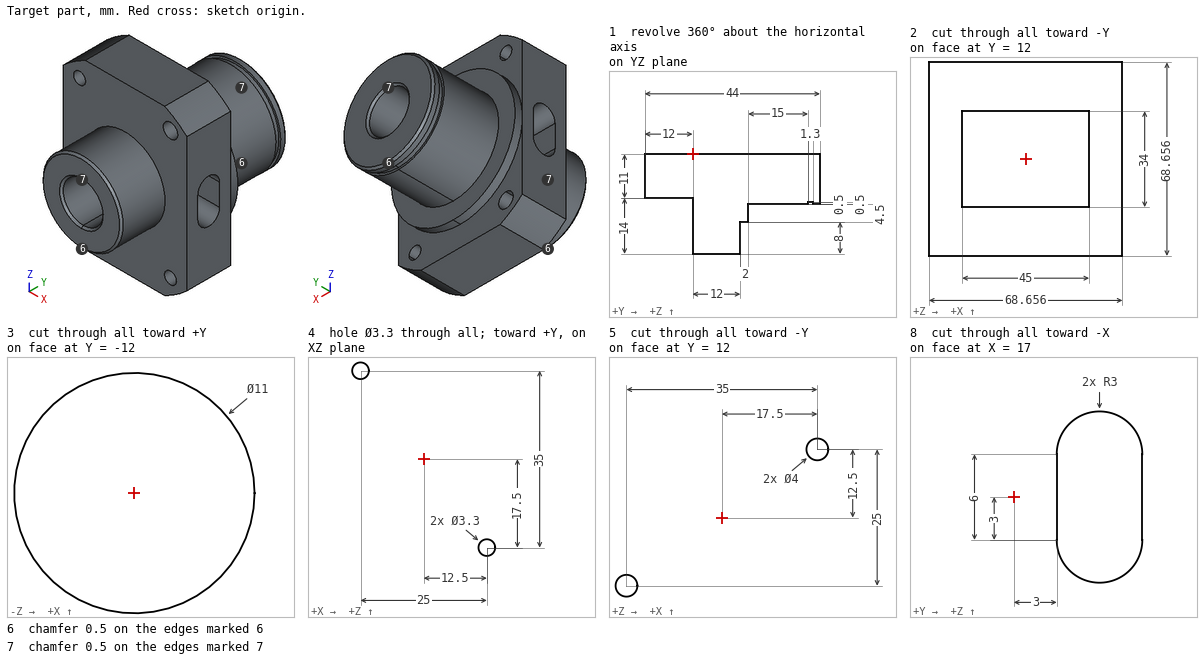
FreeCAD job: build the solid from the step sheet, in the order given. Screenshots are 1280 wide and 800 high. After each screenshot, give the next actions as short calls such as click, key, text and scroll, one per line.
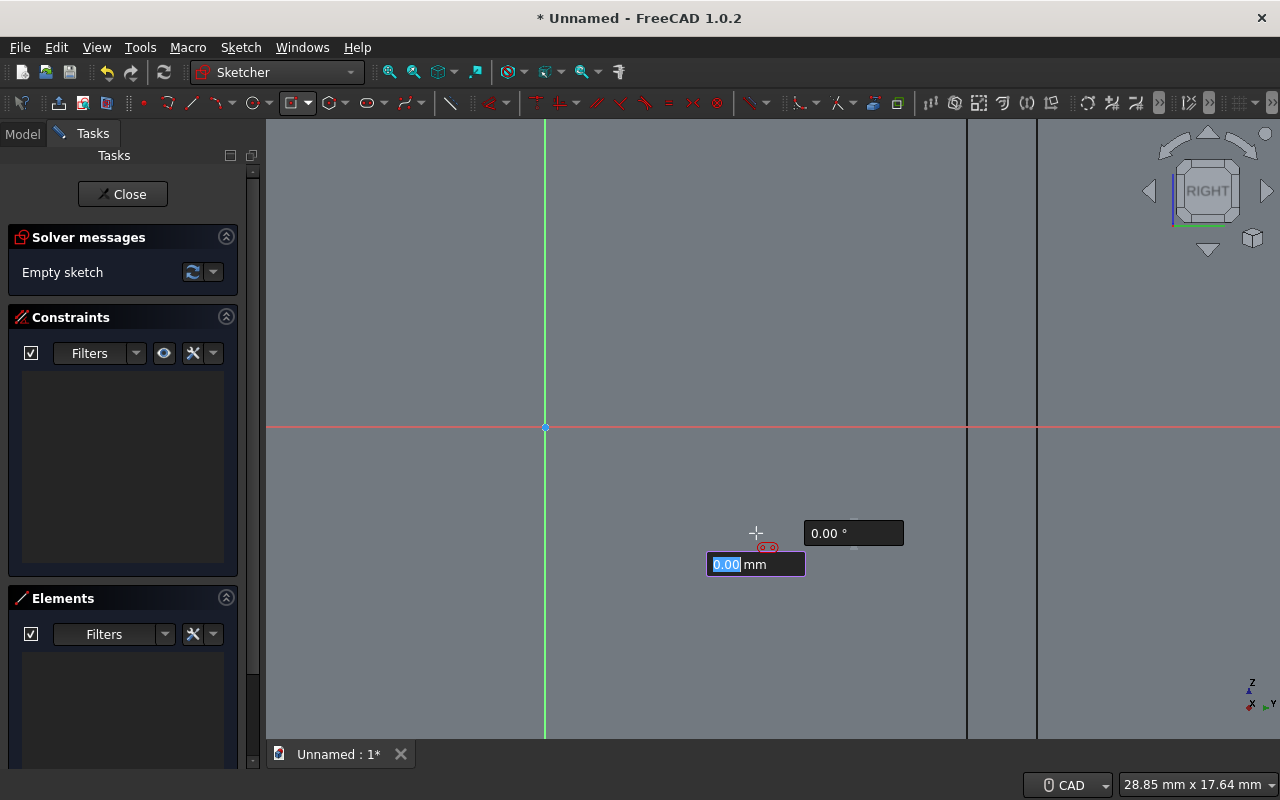
click(756, 322)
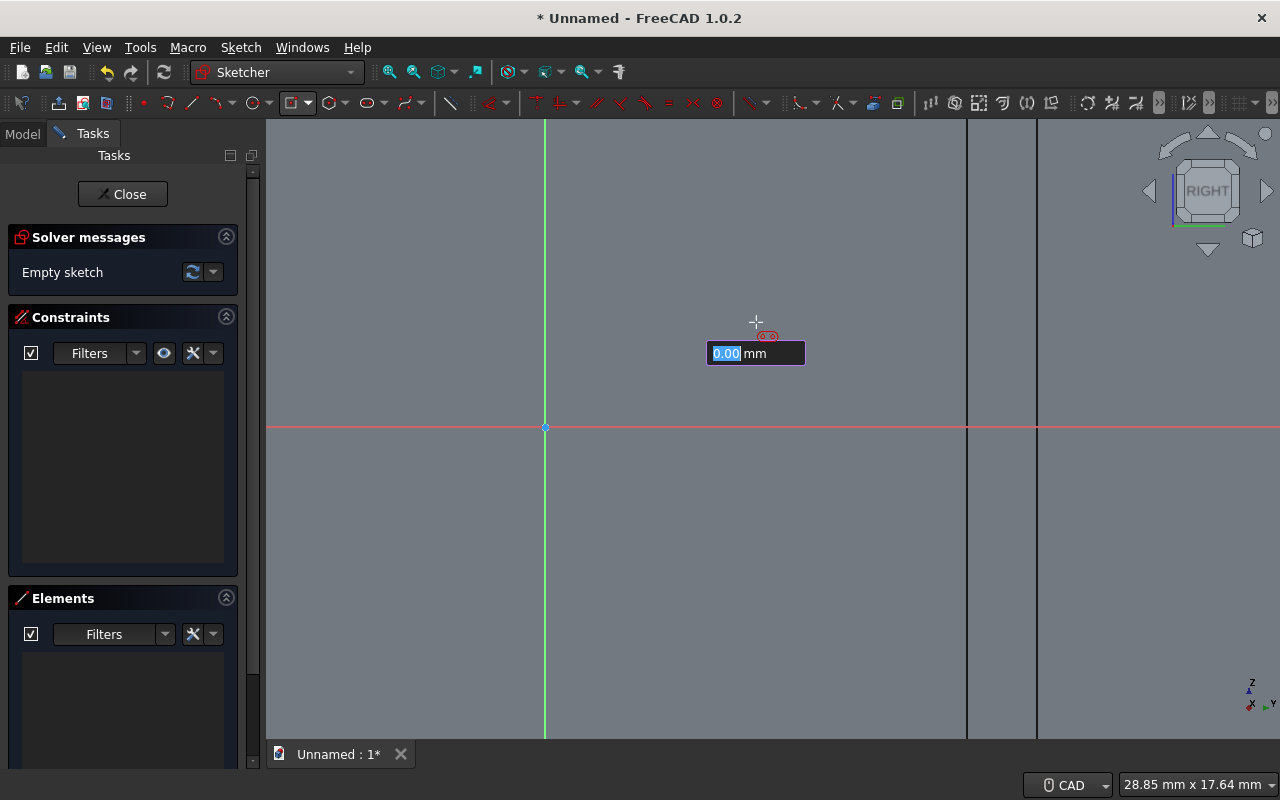
click(862, 459)
key(Escape)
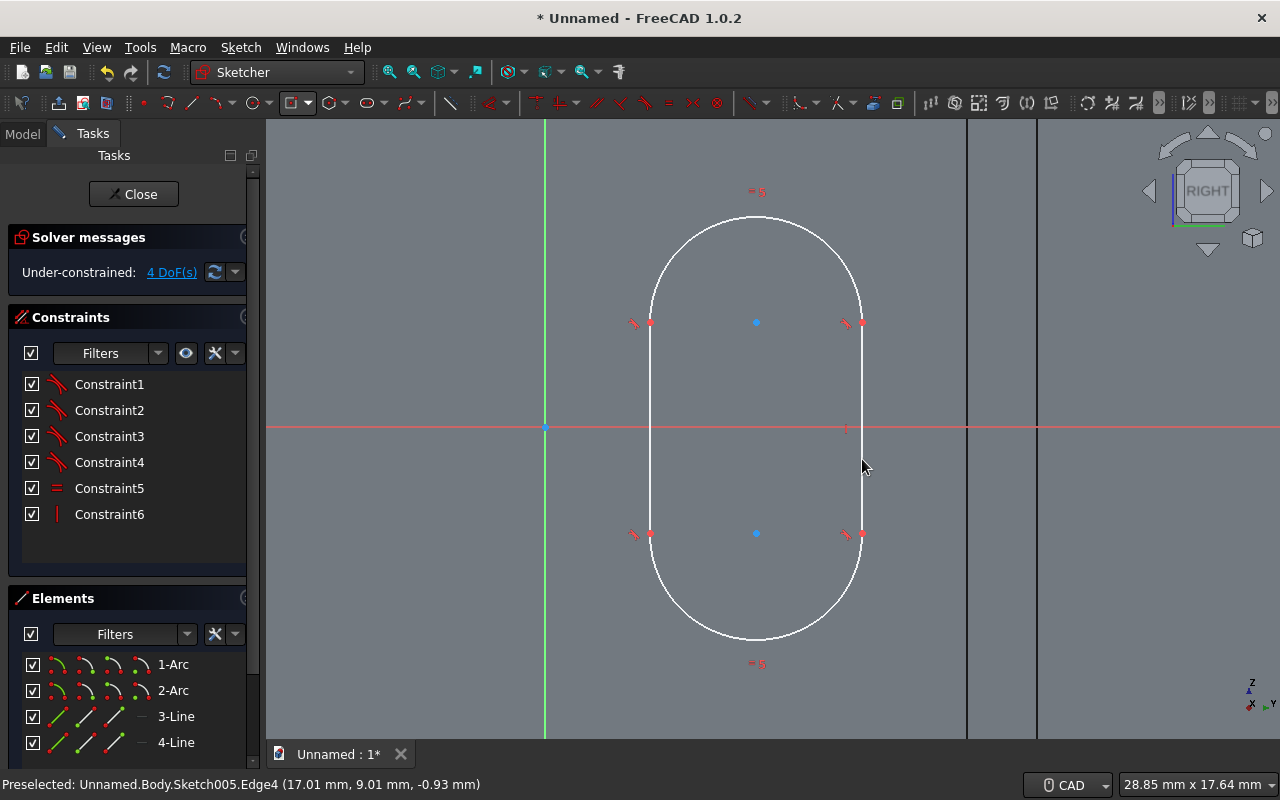
key(d)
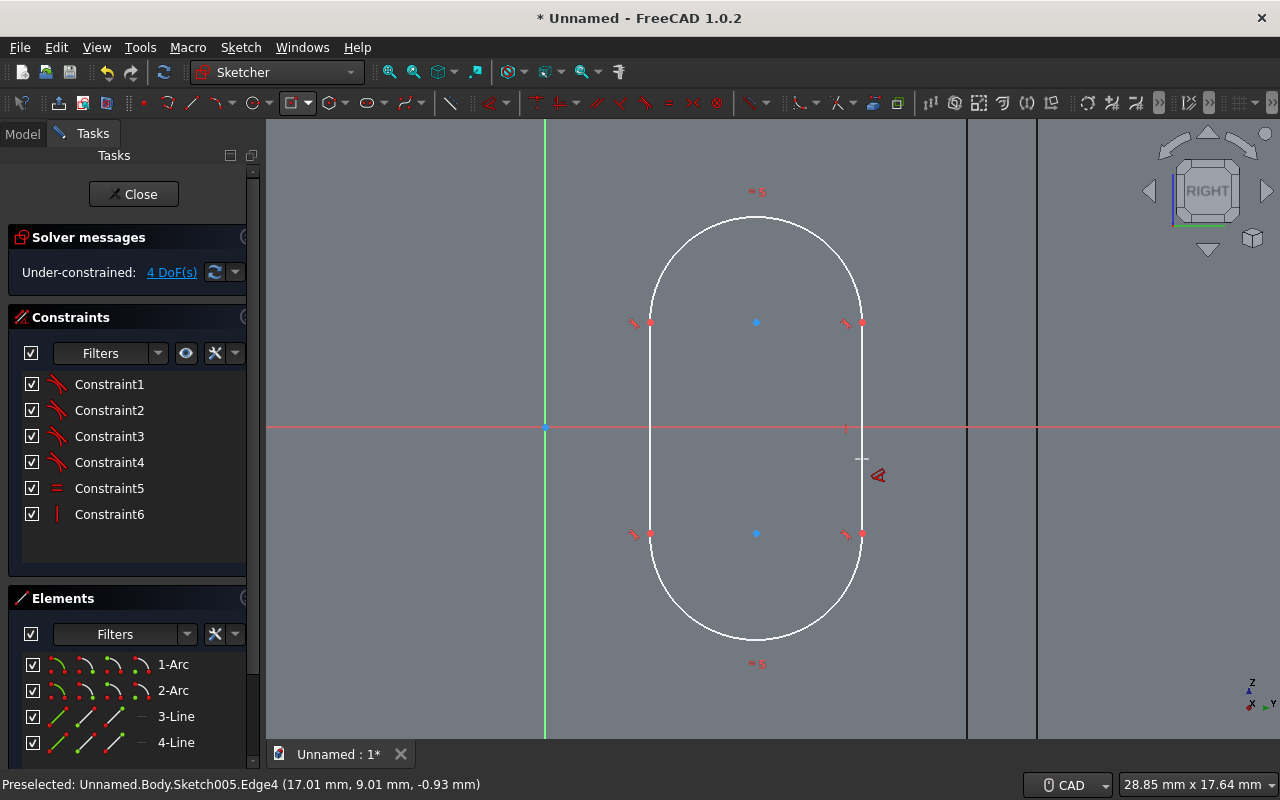
click(694, 620)
click(675, 646)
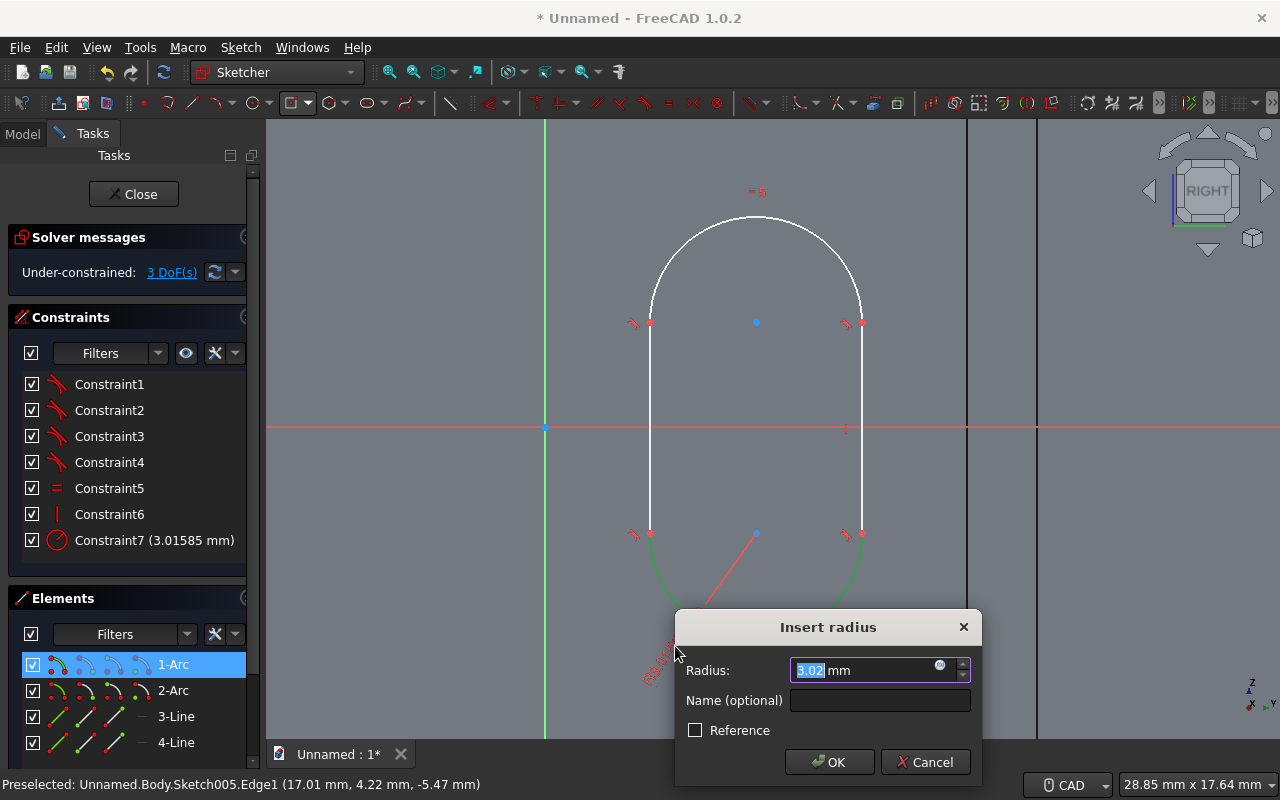
text(3)
key(Return)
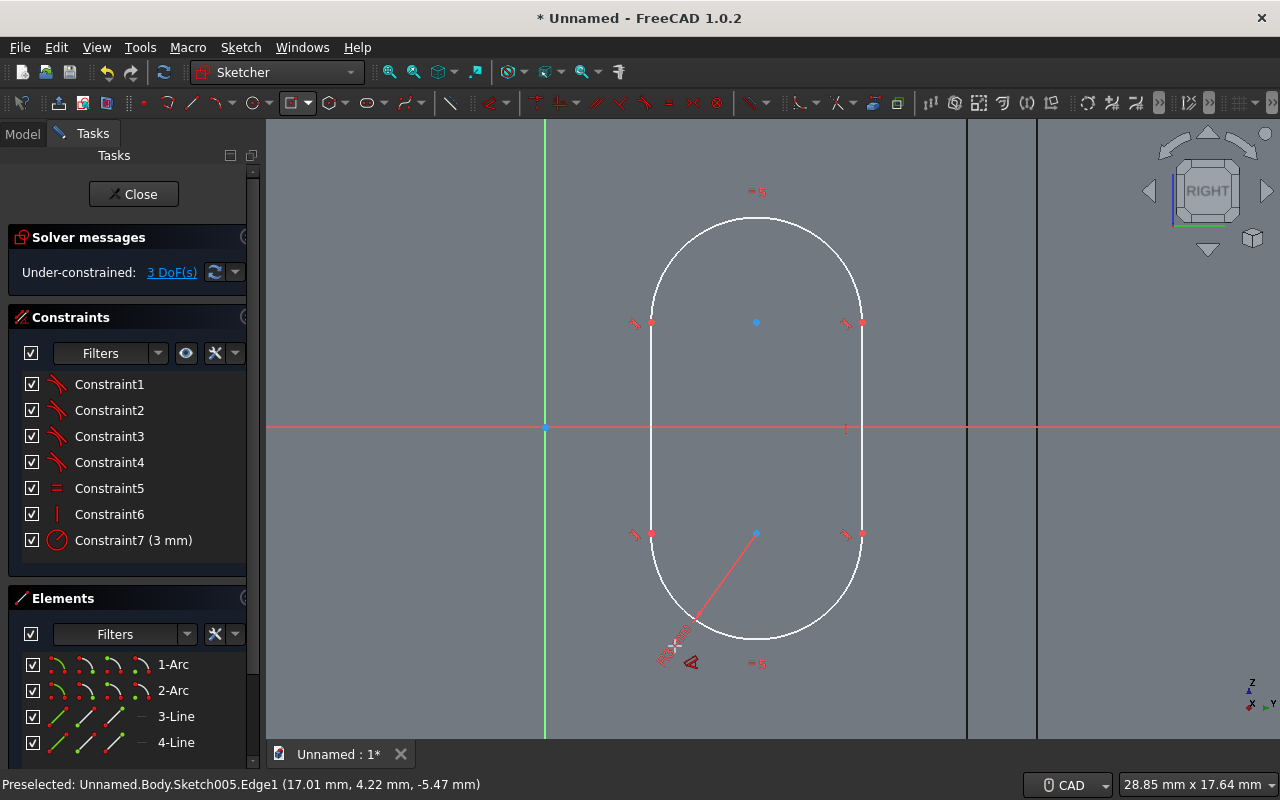
click(651, 471)
click(617, 380)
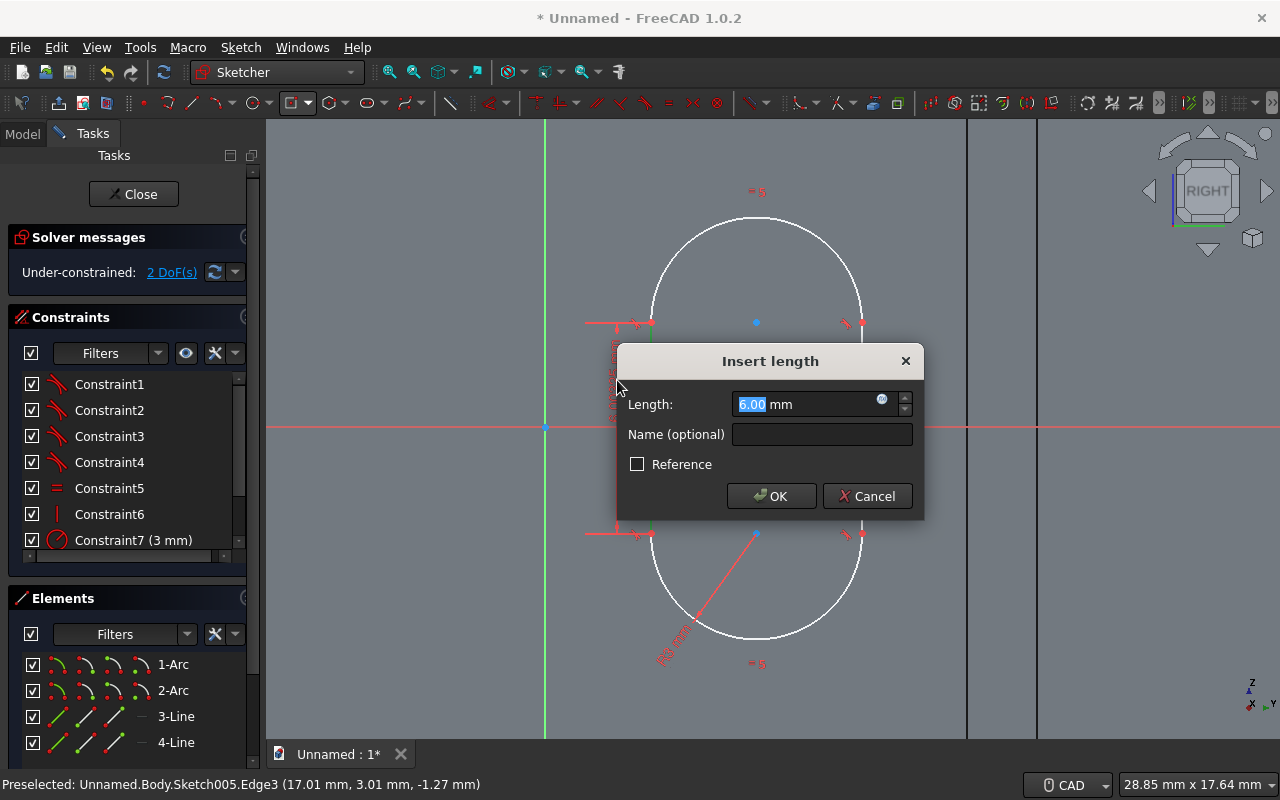
text(6)
key(Return)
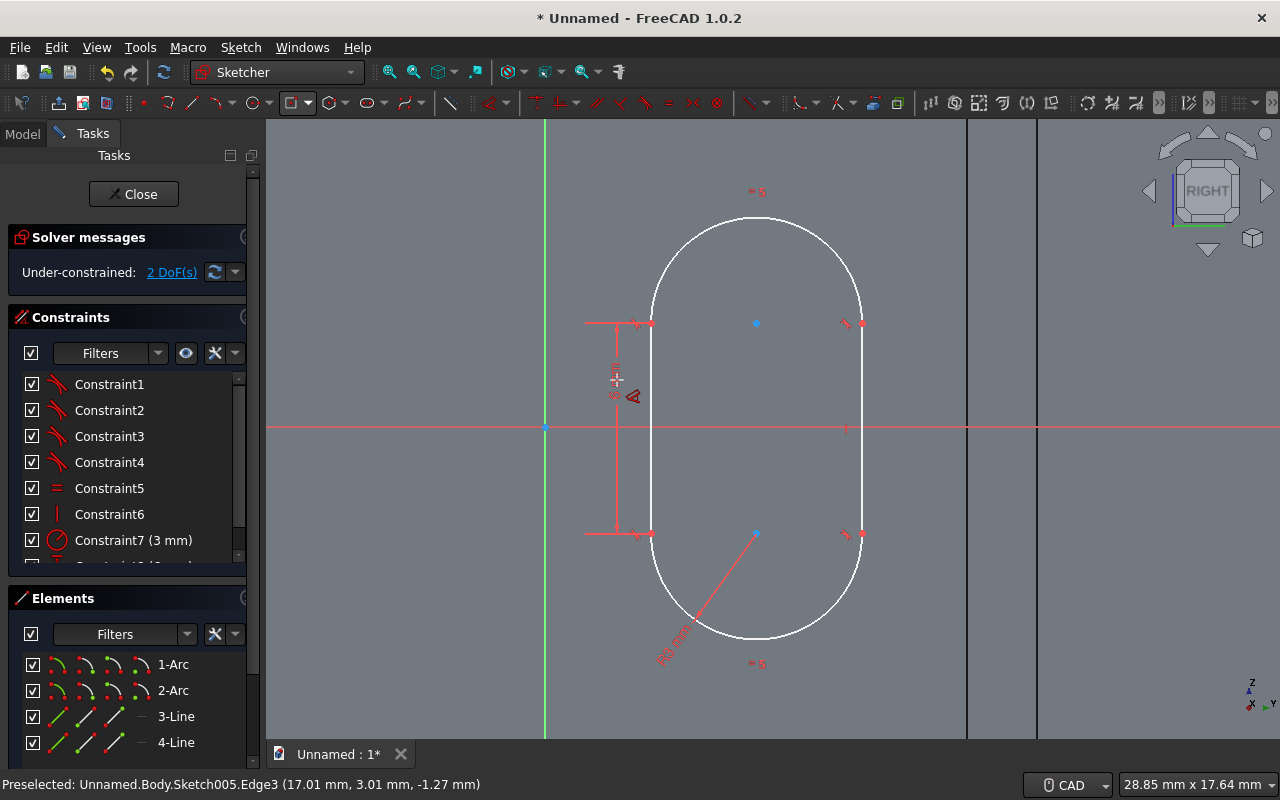
click(651, 534)
click(598, 568)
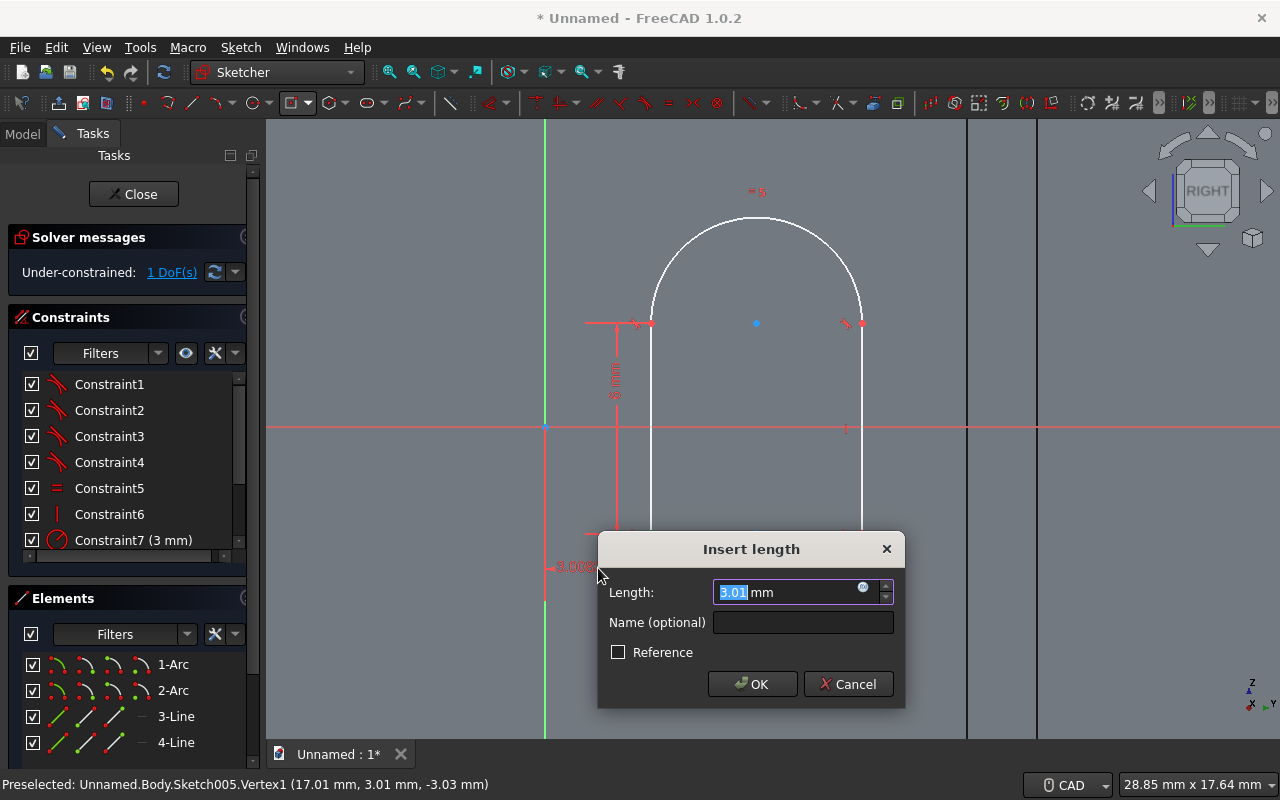
text(3)
key(Return)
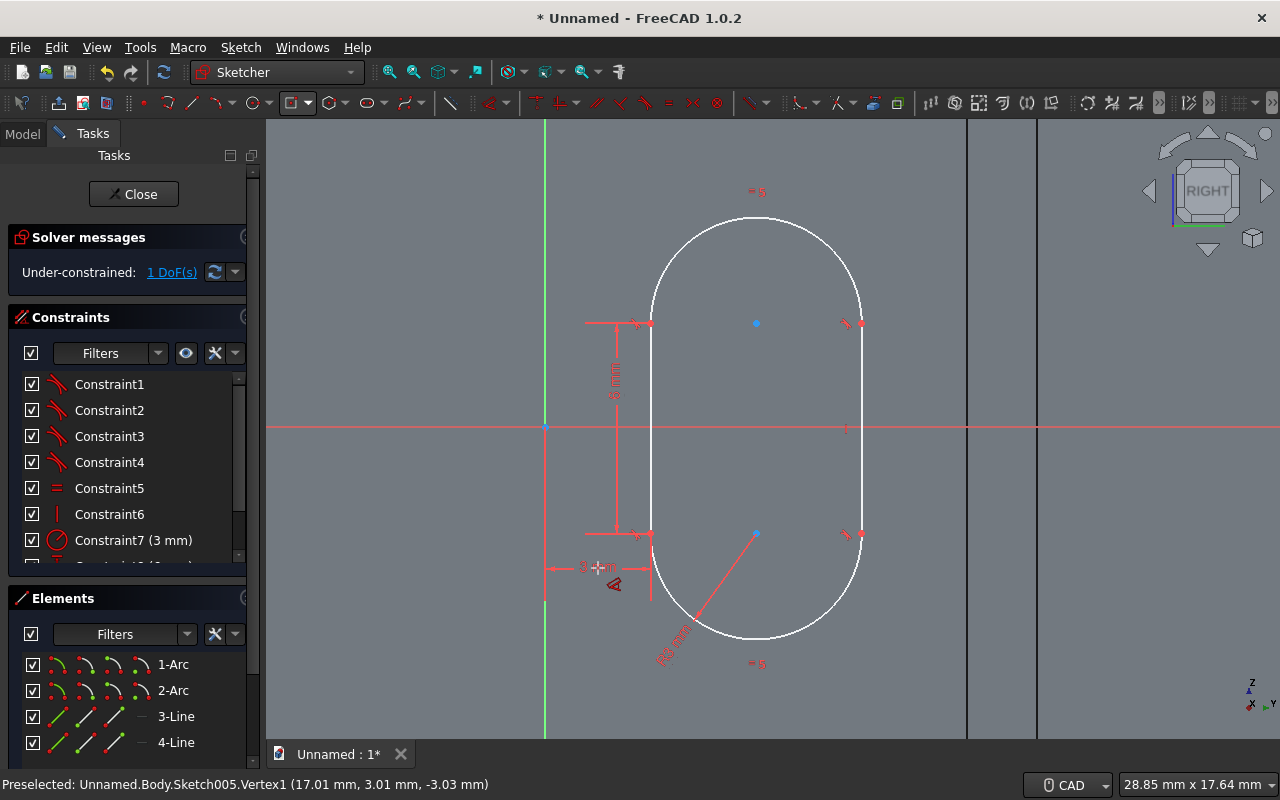
click(651, 534)
click(511, 481)